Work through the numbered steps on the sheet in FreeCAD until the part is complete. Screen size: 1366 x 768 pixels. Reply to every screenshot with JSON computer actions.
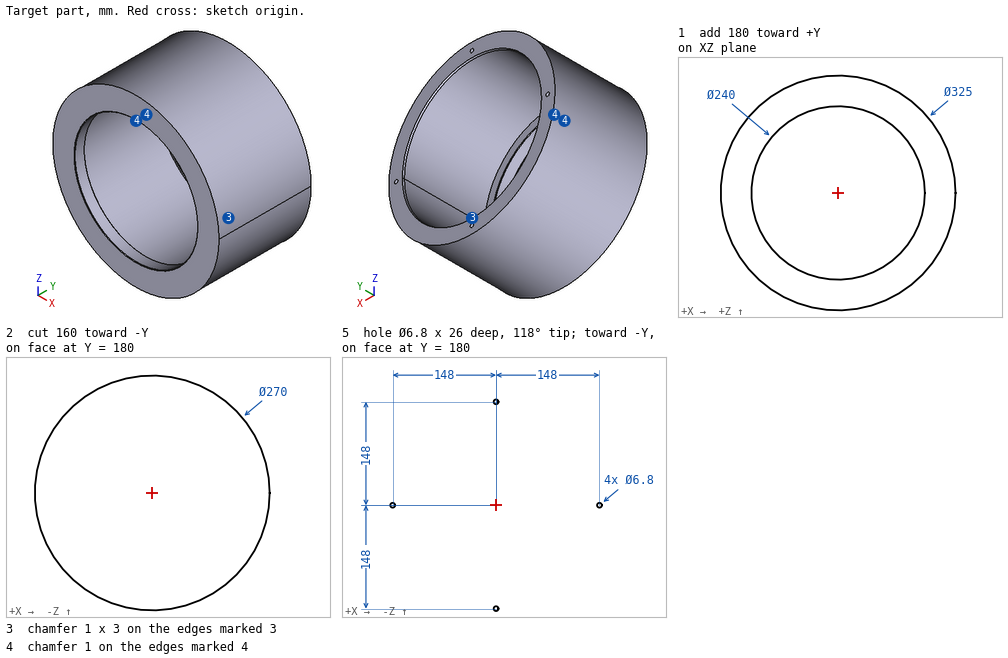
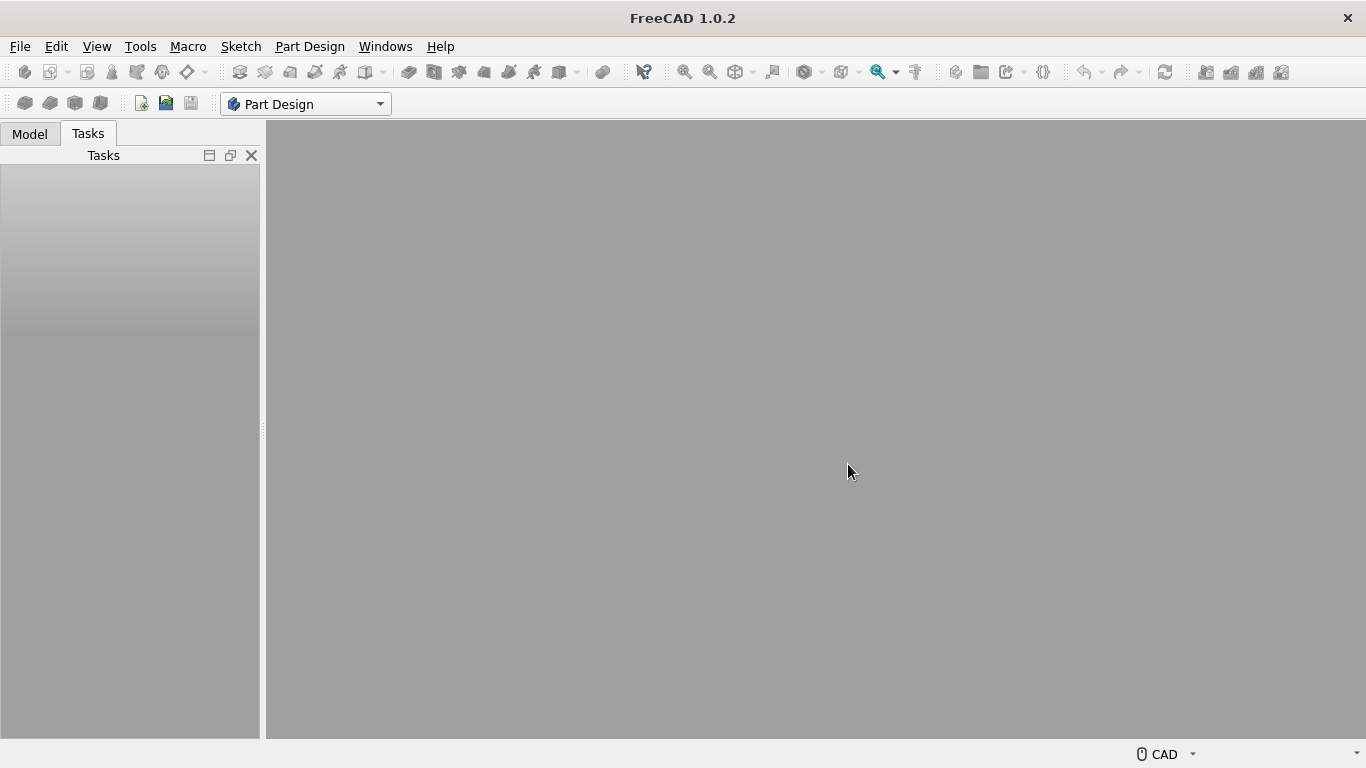
{"action": "left_click", "coordinate": [141, 104]}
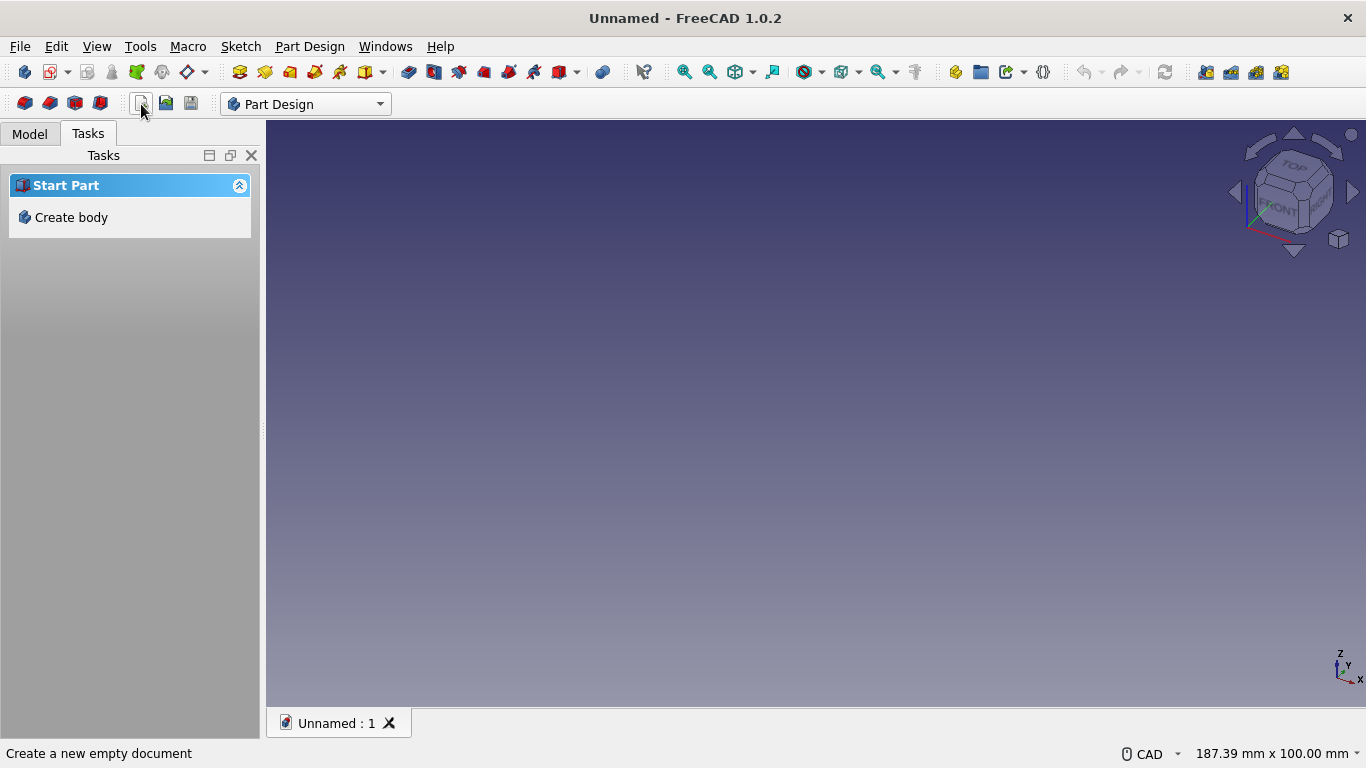
{"action": "left_click", "coordinate": [50, 72]}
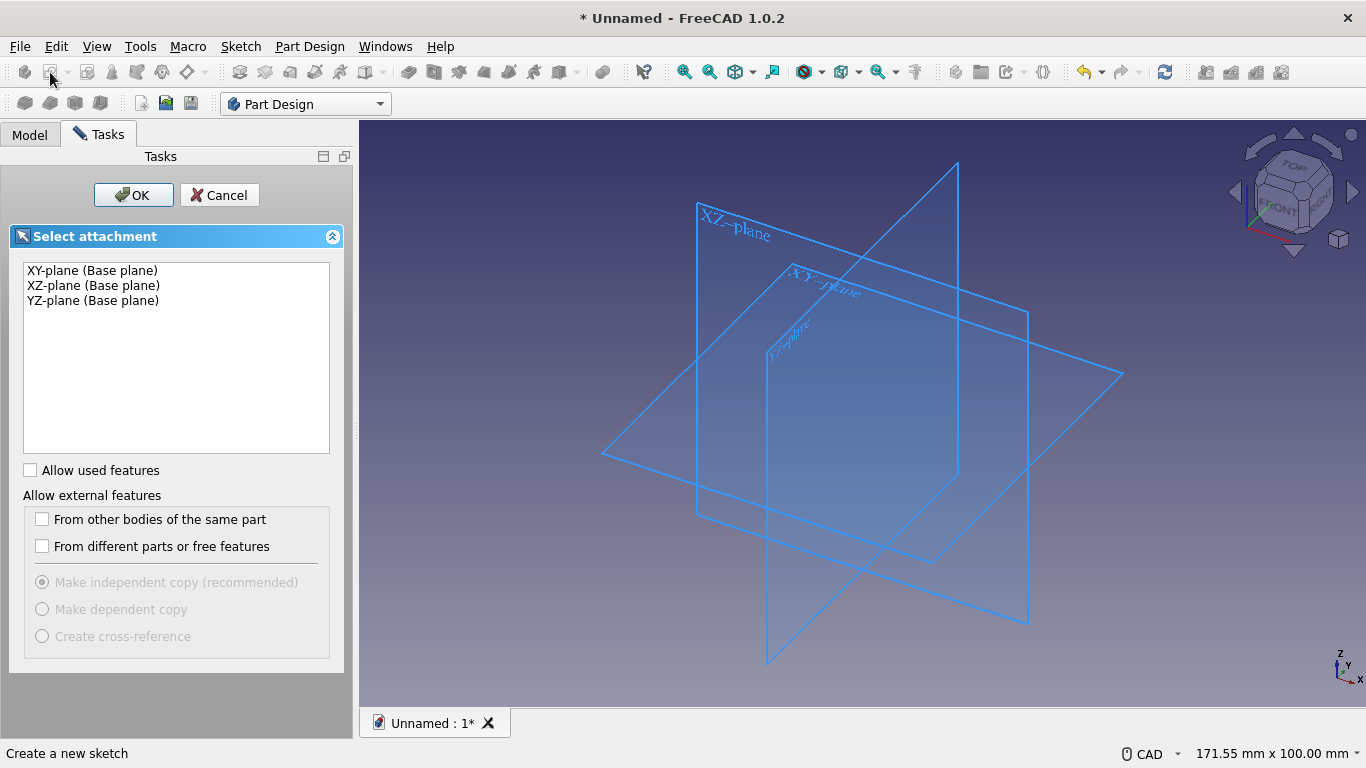
{"action": "left_click", "coordinate": [84, 286]}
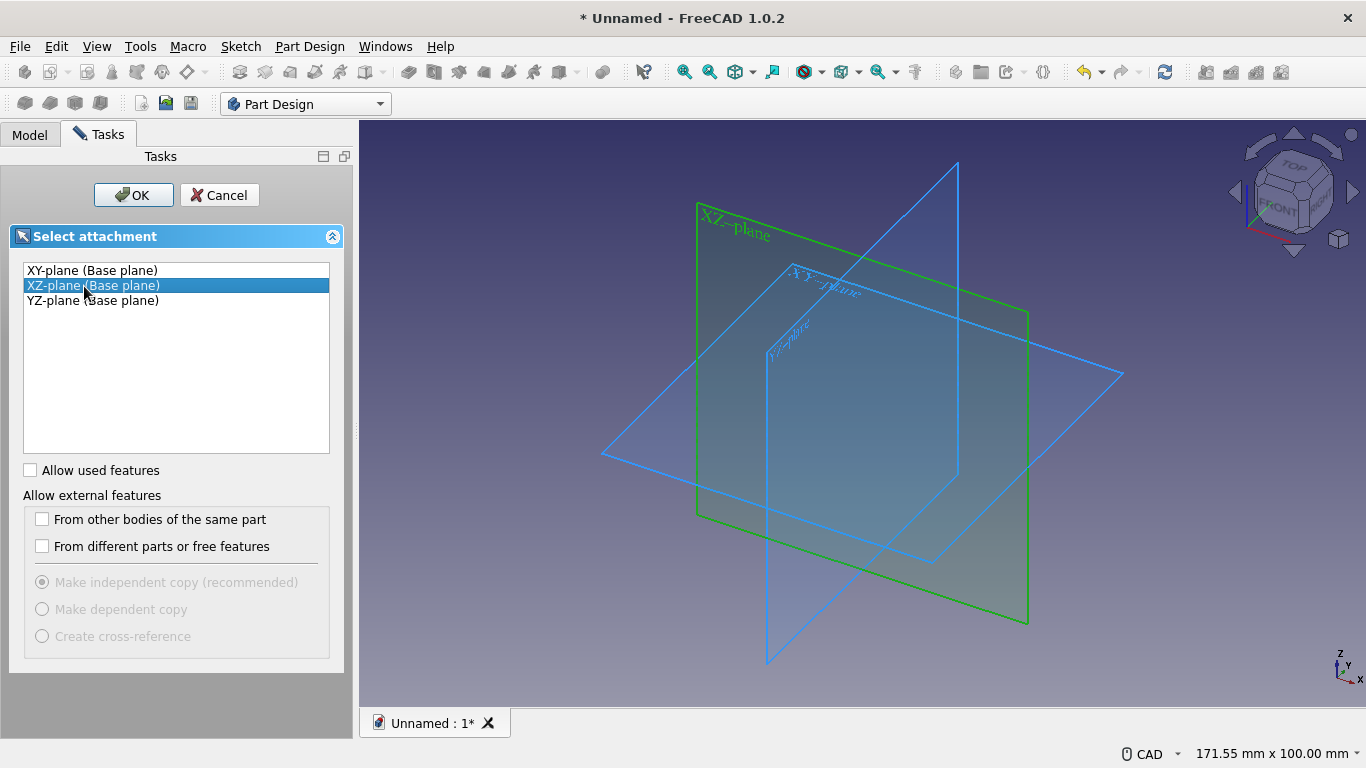
{"action": "left_click", "coordinate": [134, 195]}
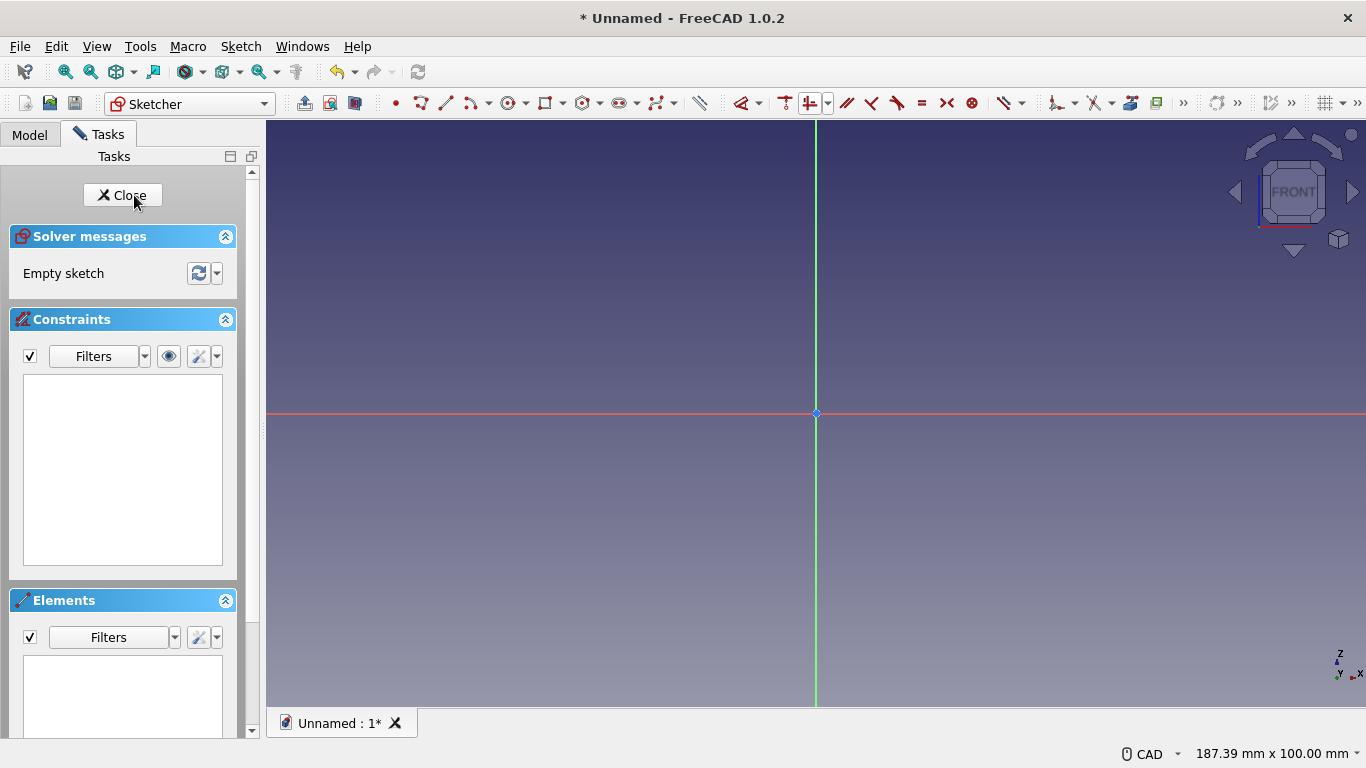
{"action": "scroll", "coordinate": [730, 414], "scroll_direction": "down", "scroll_amount": 8}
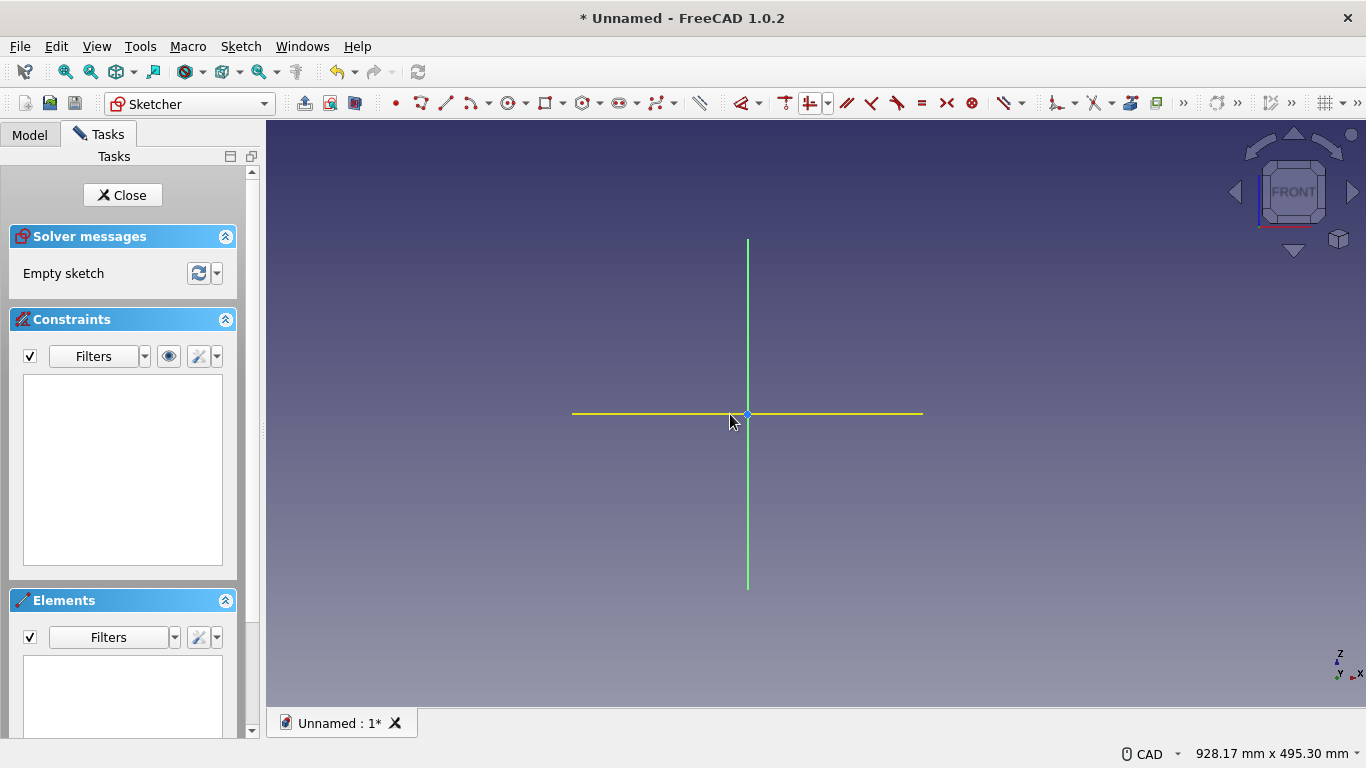
{"action": "key", "text": "g c"}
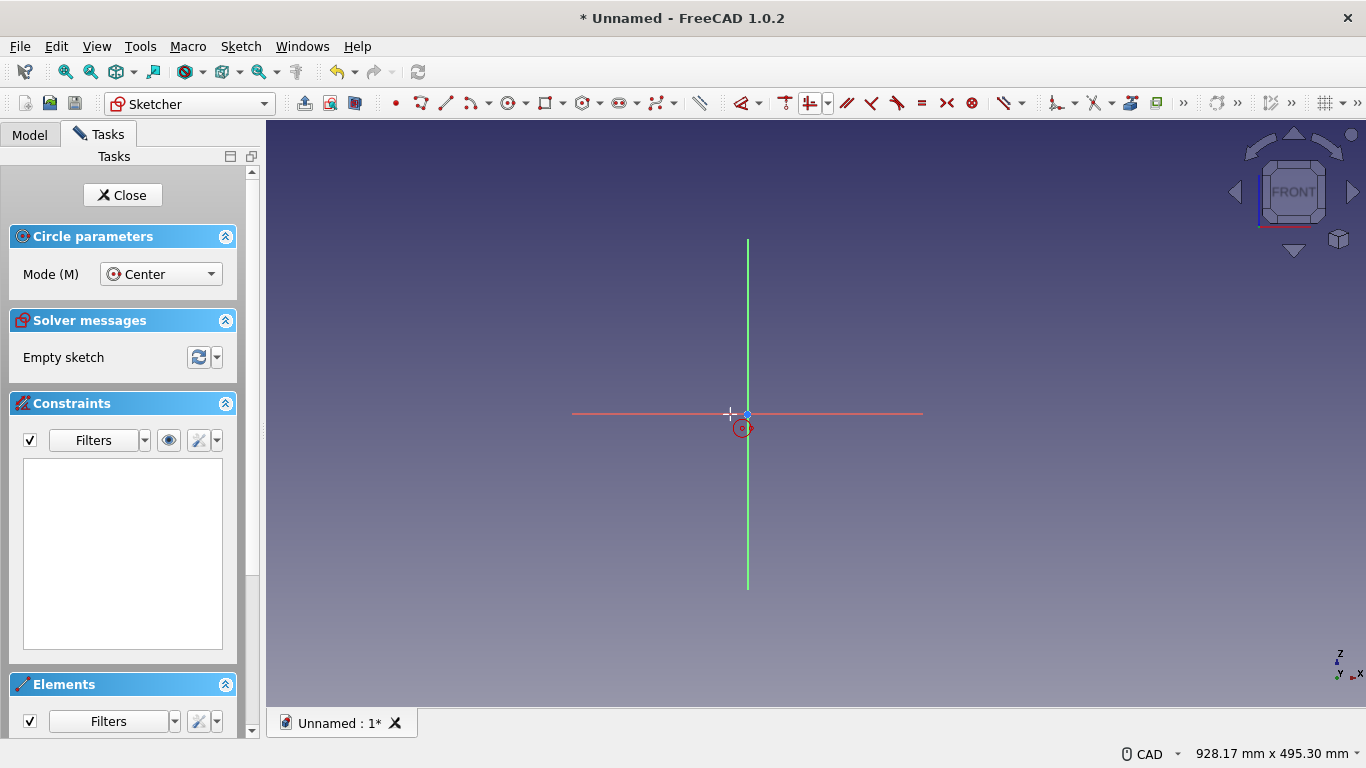
{"action": "left_click", "coordinate": [748, 414]}
{"action": "mouse_move", "coordinate": [884, 278]}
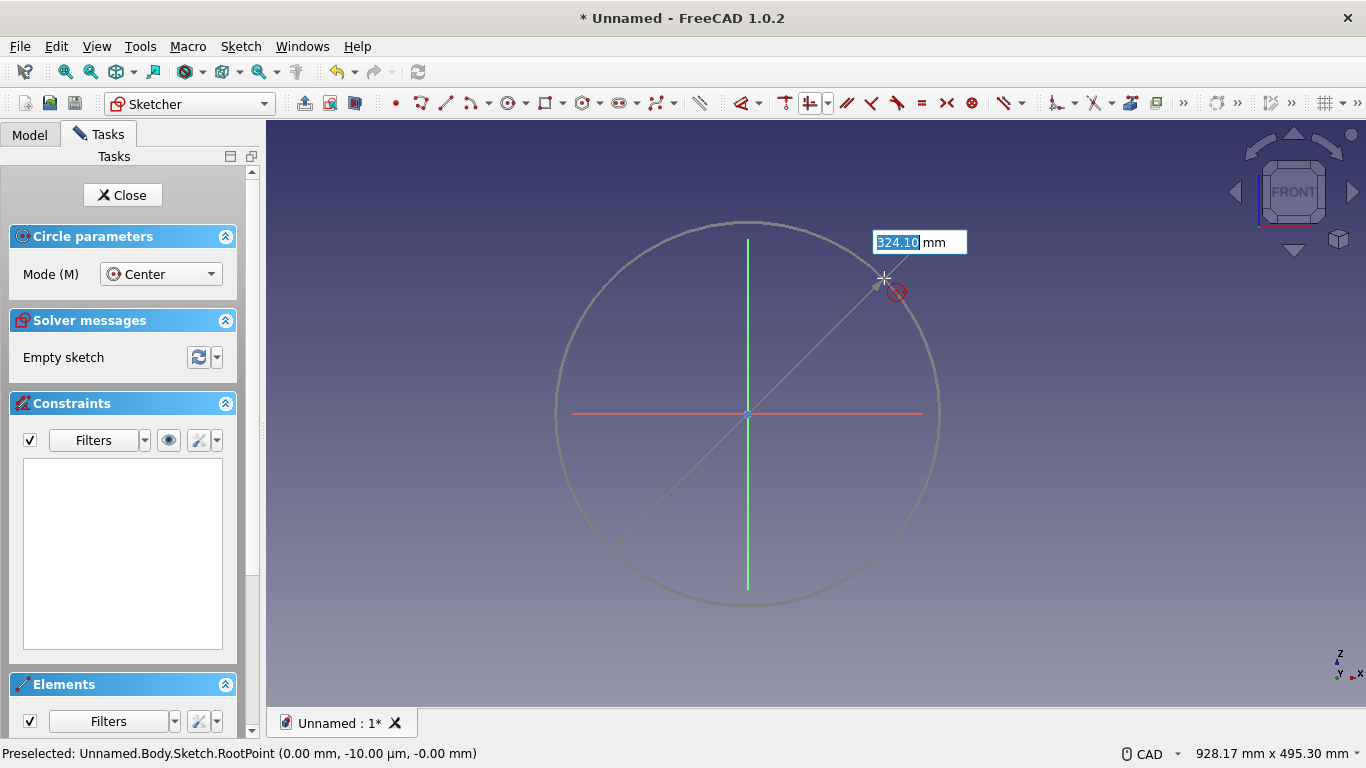
{"action": "type", "text": "325"}
{"action": "key", "text": "Return"}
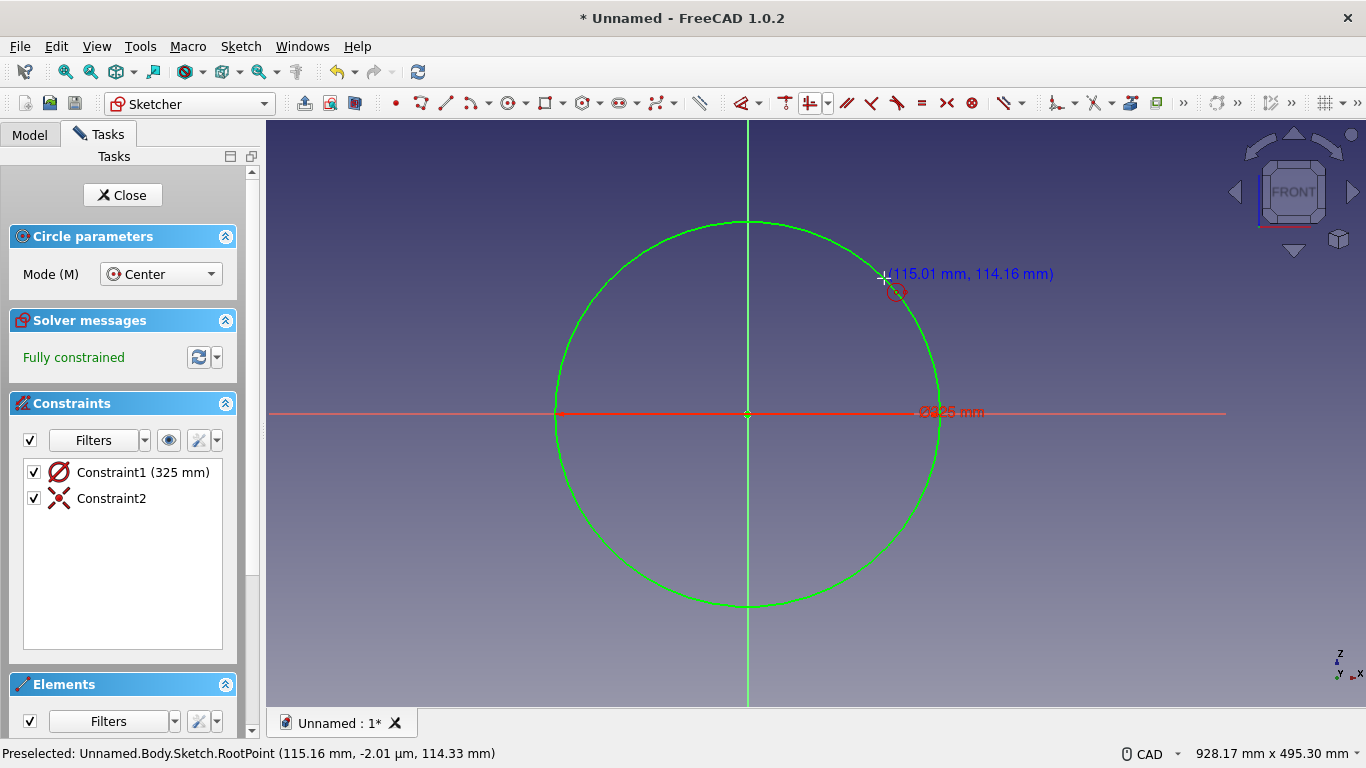
{"action": "left_click", "coordinate": [748, 414]}
{"action": "mouse_move", "coordinate": [848, 314]}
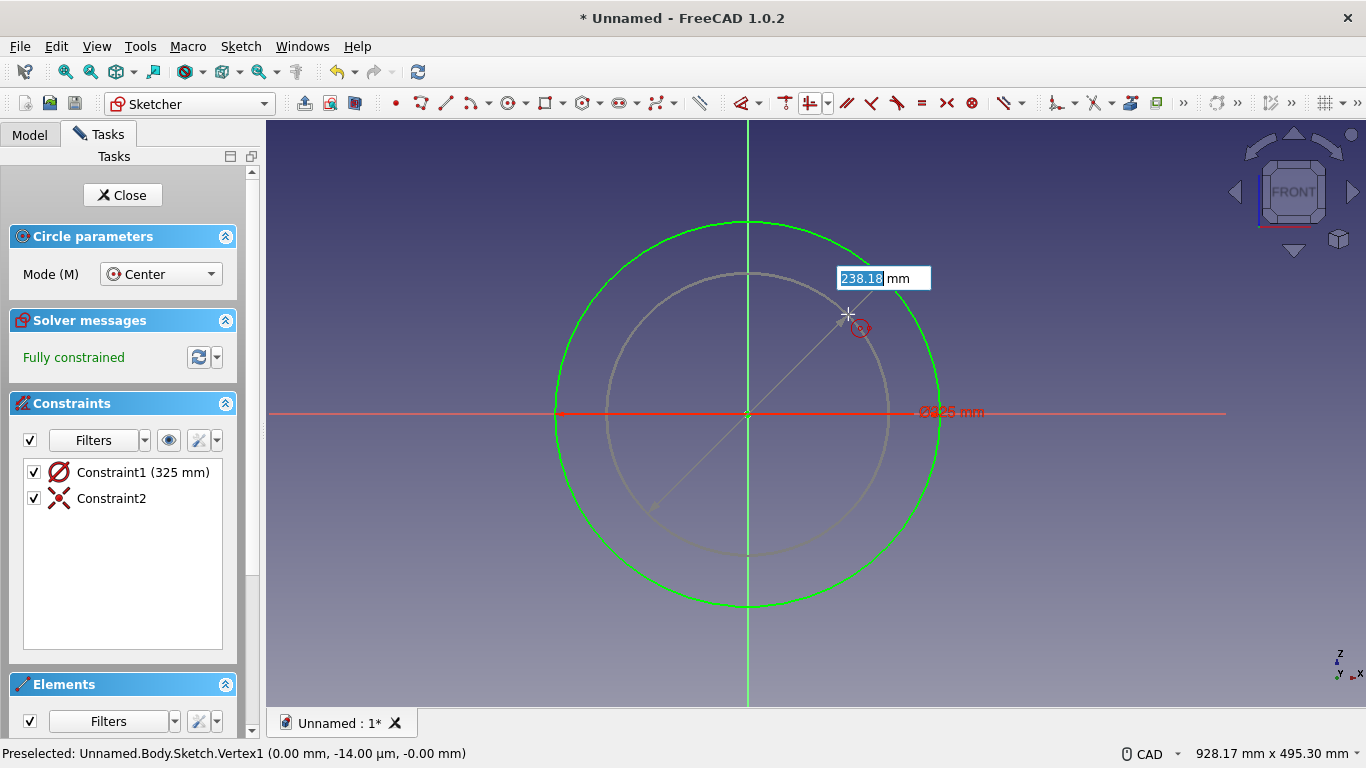
{"action": "type", "text": "240"}
{"action": "key", "text": "Return"}
{"action": "key", "text": "Escape"}